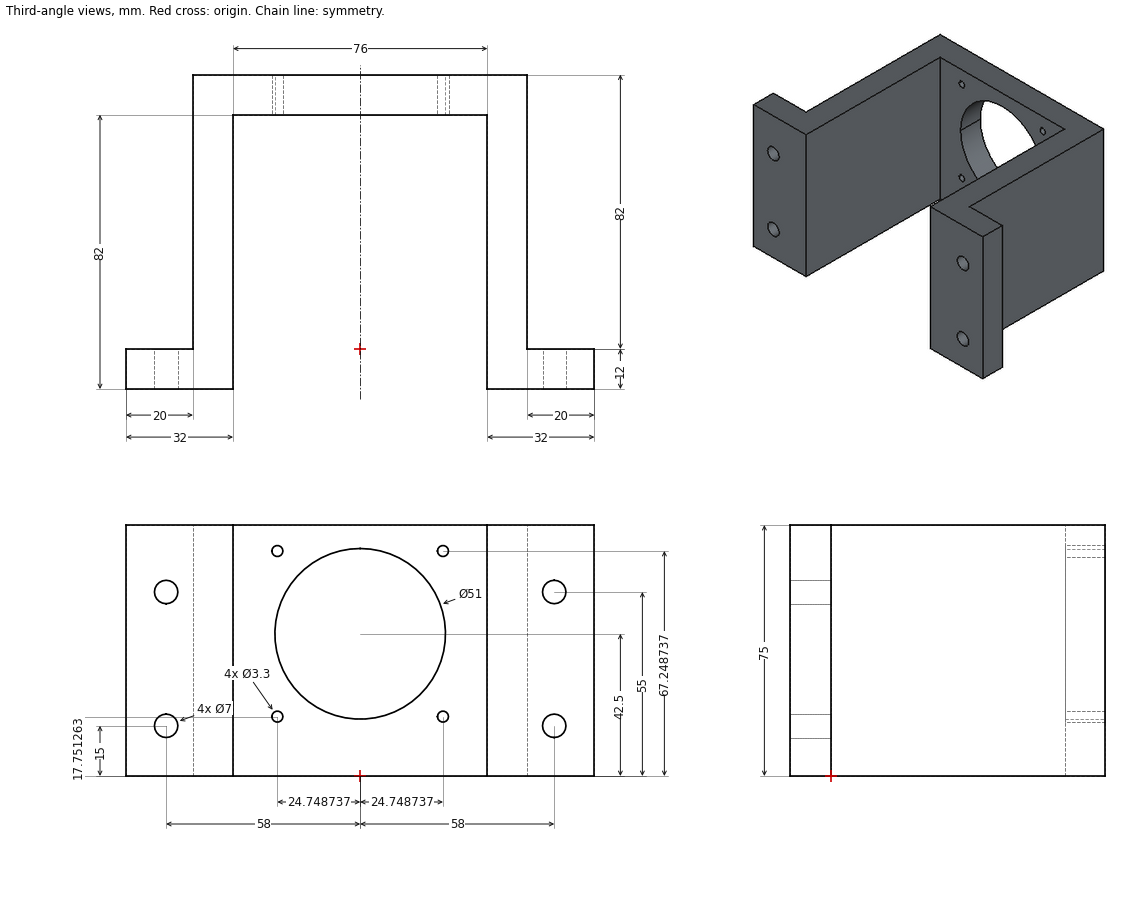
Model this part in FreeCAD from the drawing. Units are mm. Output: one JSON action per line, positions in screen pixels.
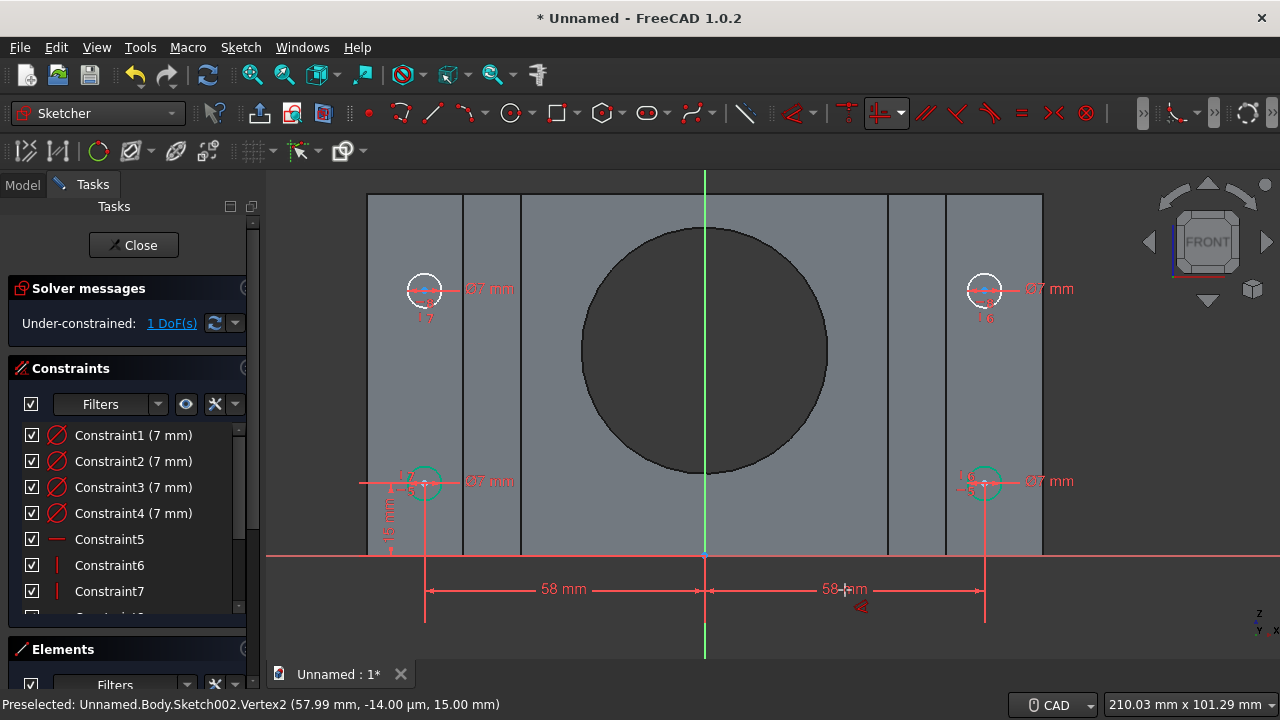
{"action": "left_click", "coordinate": [985, 291]}
{"action": "left_click", "coordinate": [1019, 423]}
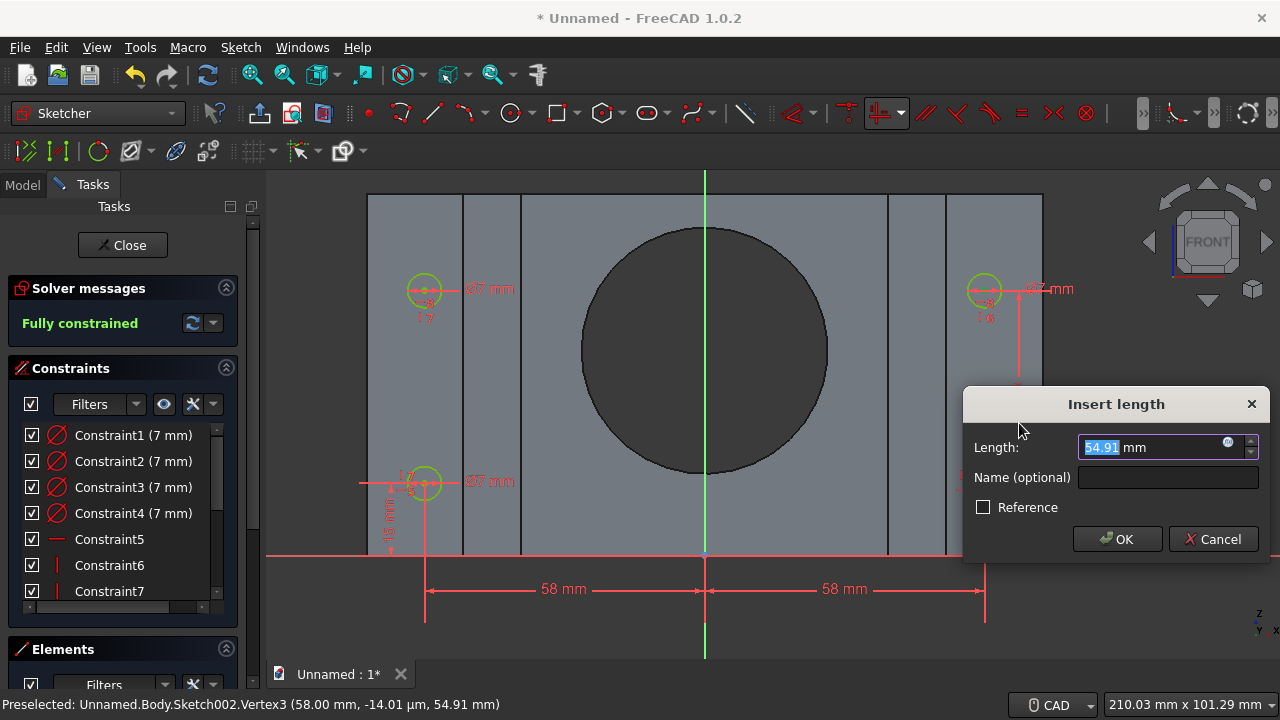
{"action": "type", "text": "55"}
{"action": "key", "text": "Return"}
{"action": "key", "text": "Escape"}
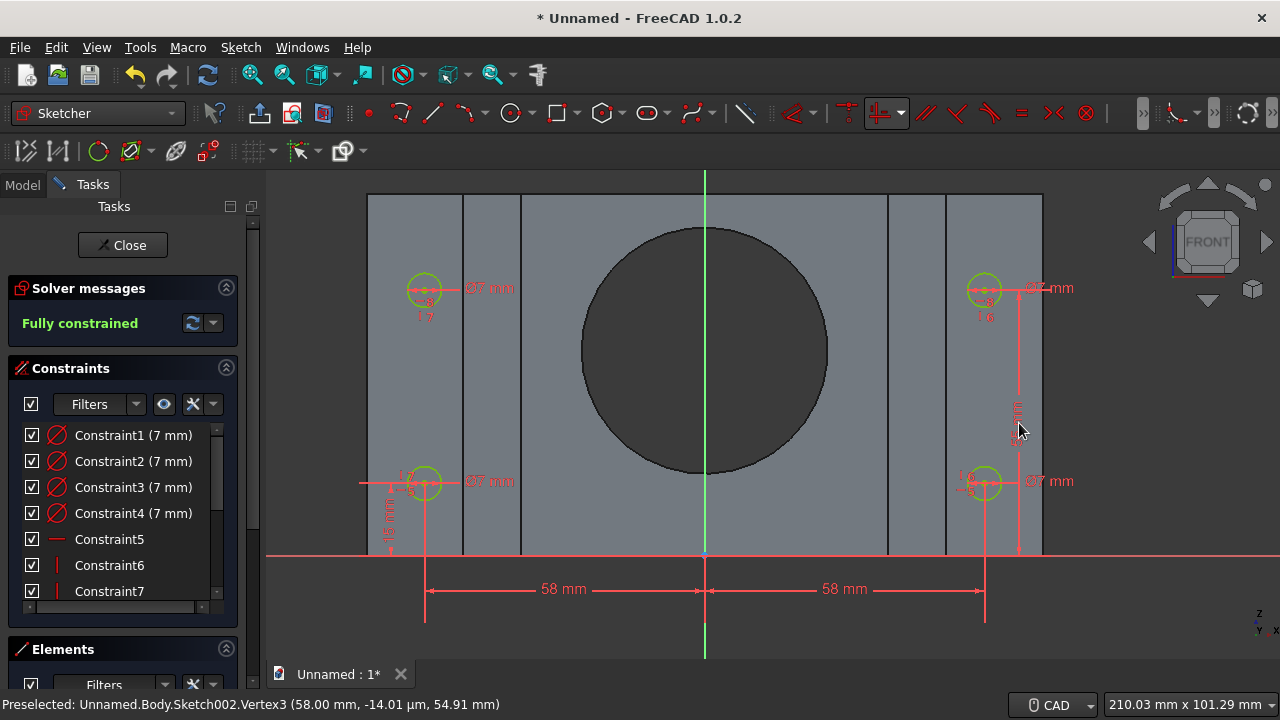
{"action": "left_click", "coordinate": [123, 245]}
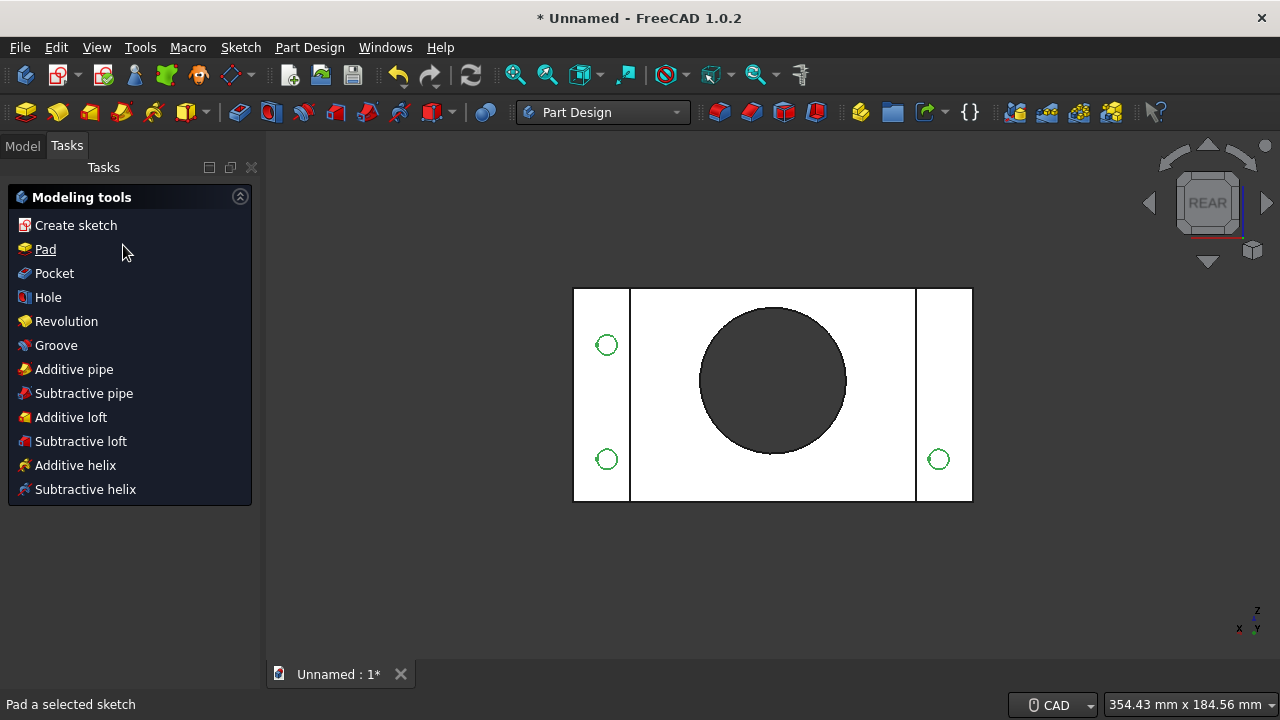
{"action": "left_click", "coordinate": [240, 112]}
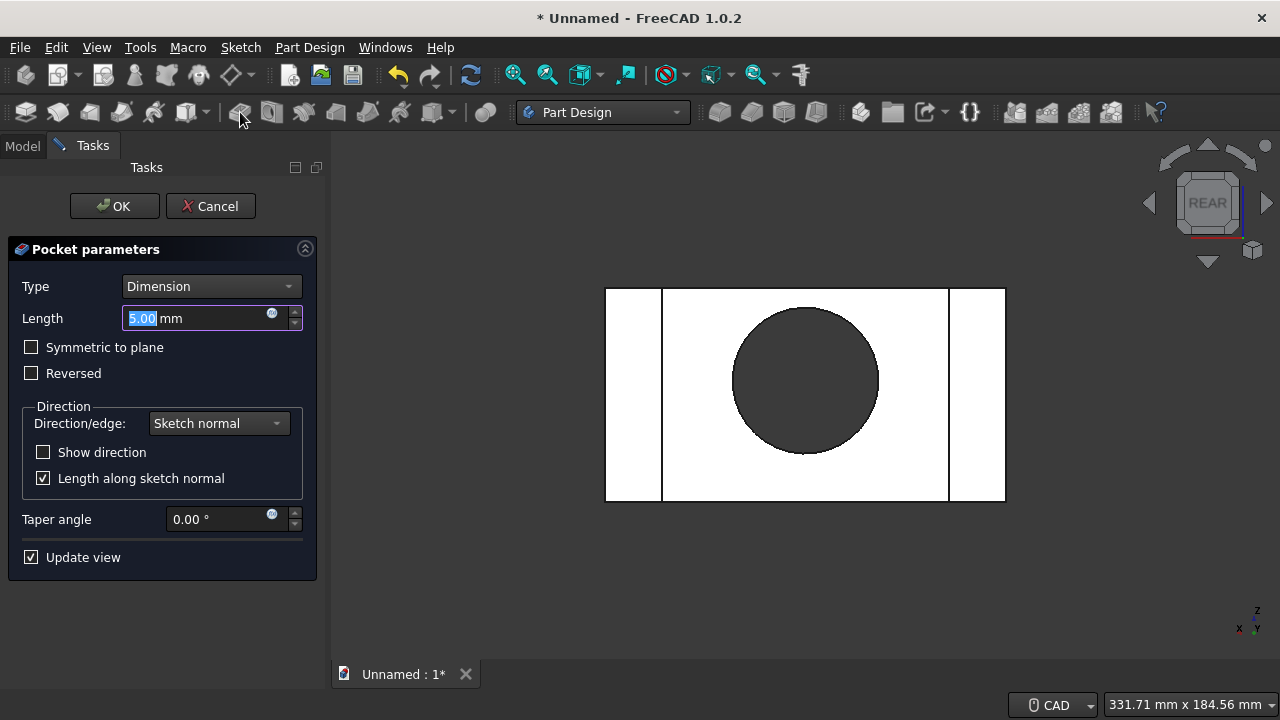
{"action": "left_click", "coordinate": [212, 286]}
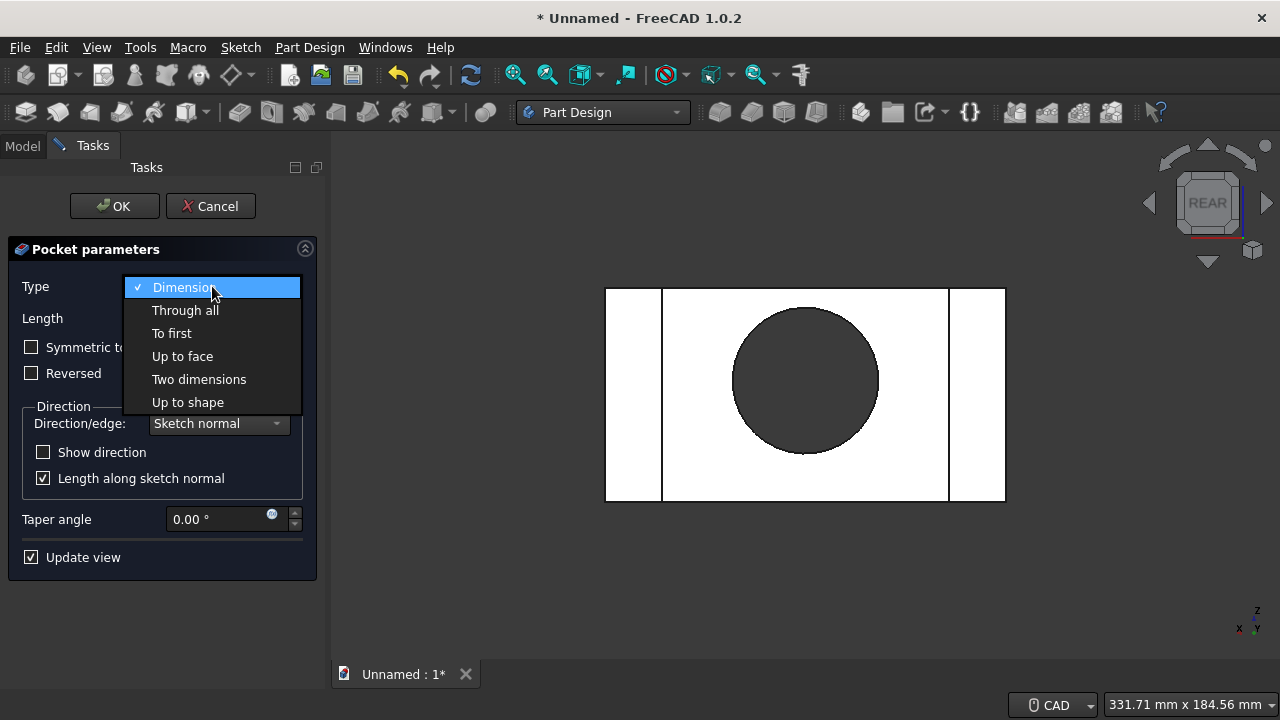
{"action": "left_click", "coordinate": [212, 310]}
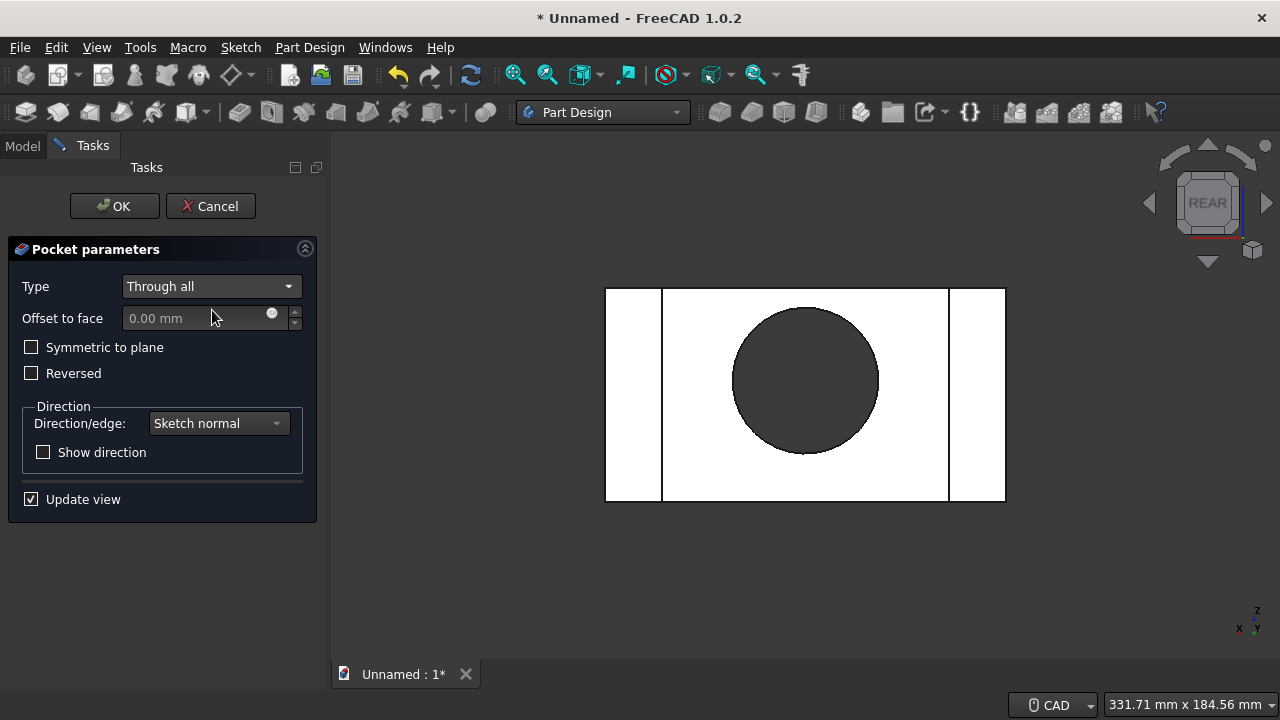
{"action": "left_click", "coordinate": [30, 373]}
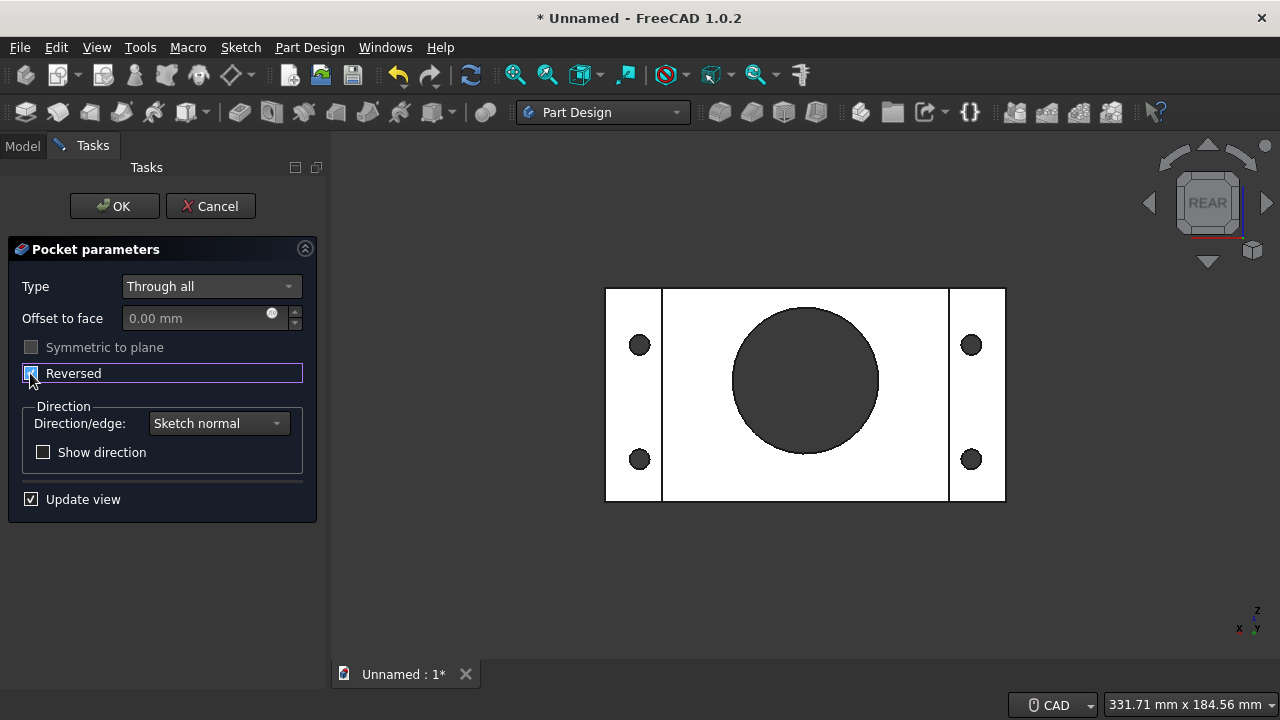
{"action": "left_click", "coordinate": [115, 206]}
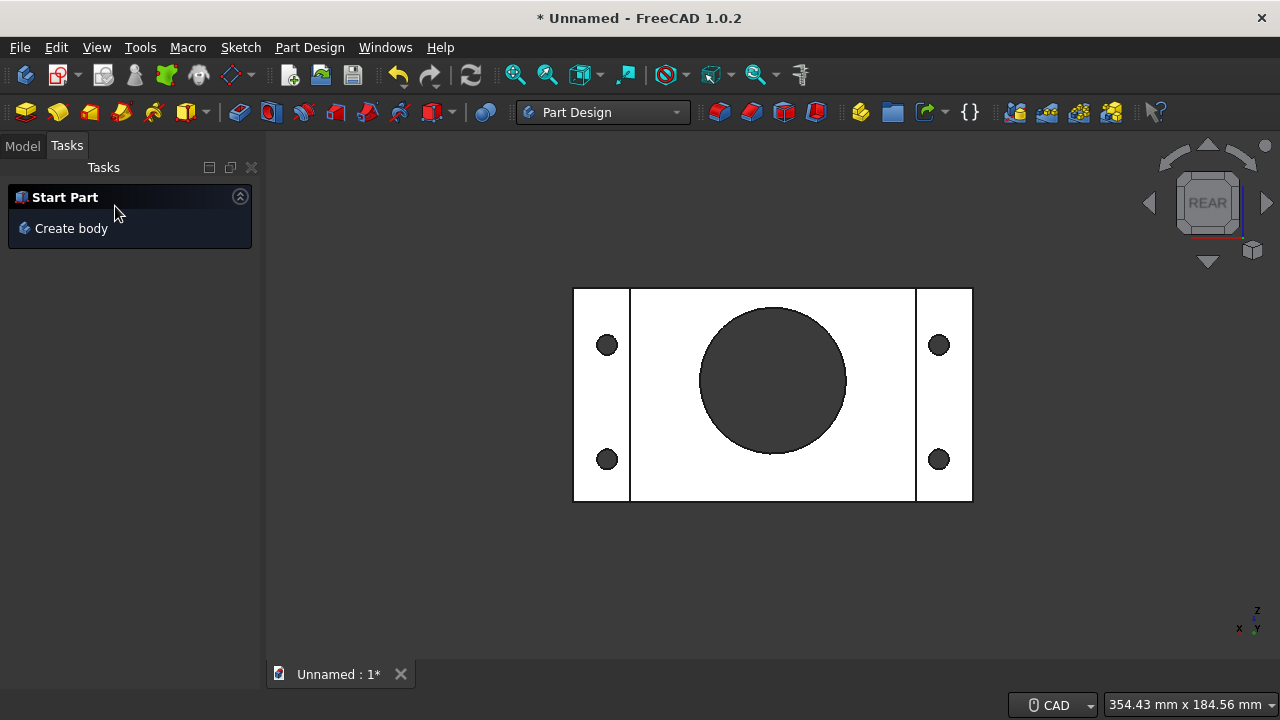
{"action": "left_click", "coordinate": [516, 76]}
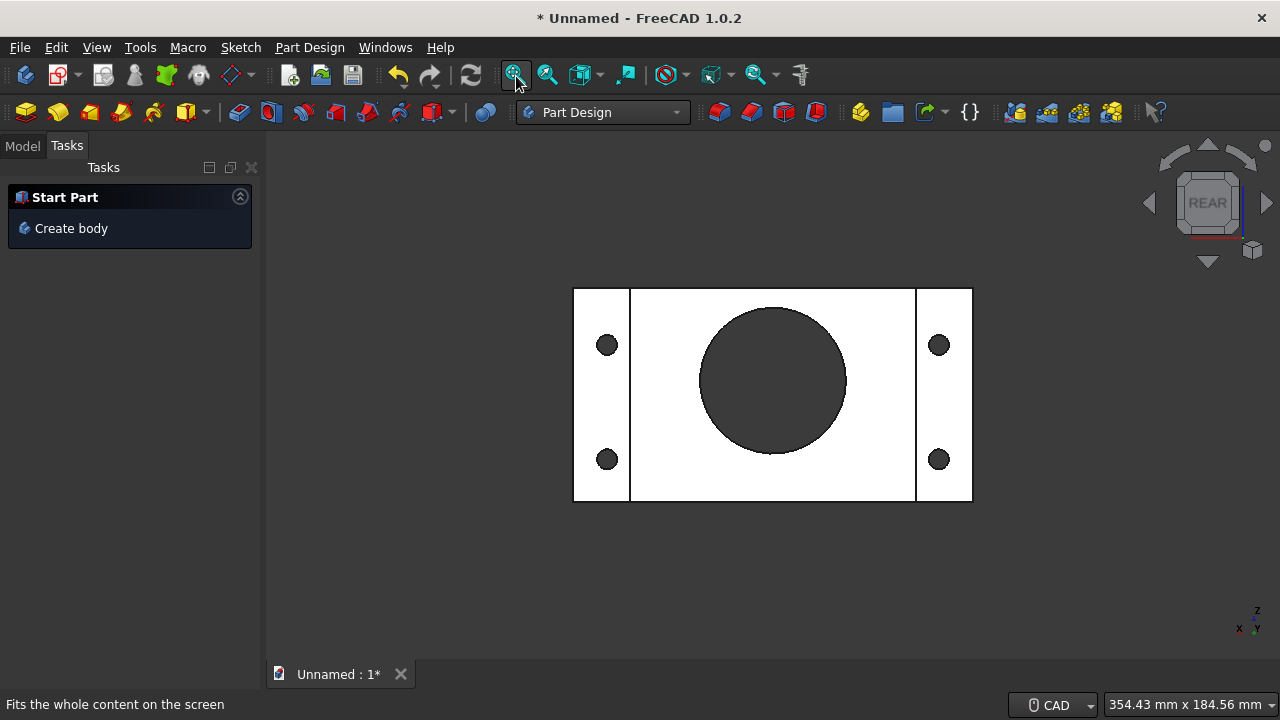
{"action": "left_click", "coordinate": [691, 455]}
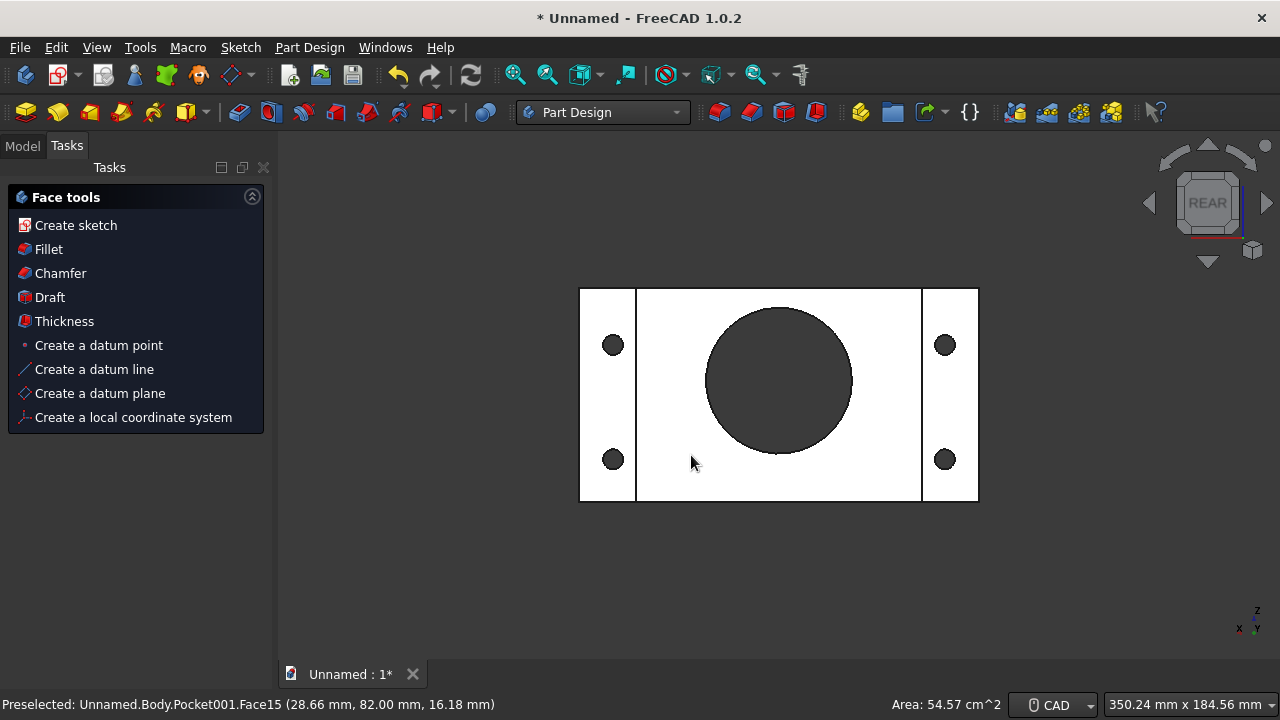
{"action": "left_click", "coordinate": [58, 76]}